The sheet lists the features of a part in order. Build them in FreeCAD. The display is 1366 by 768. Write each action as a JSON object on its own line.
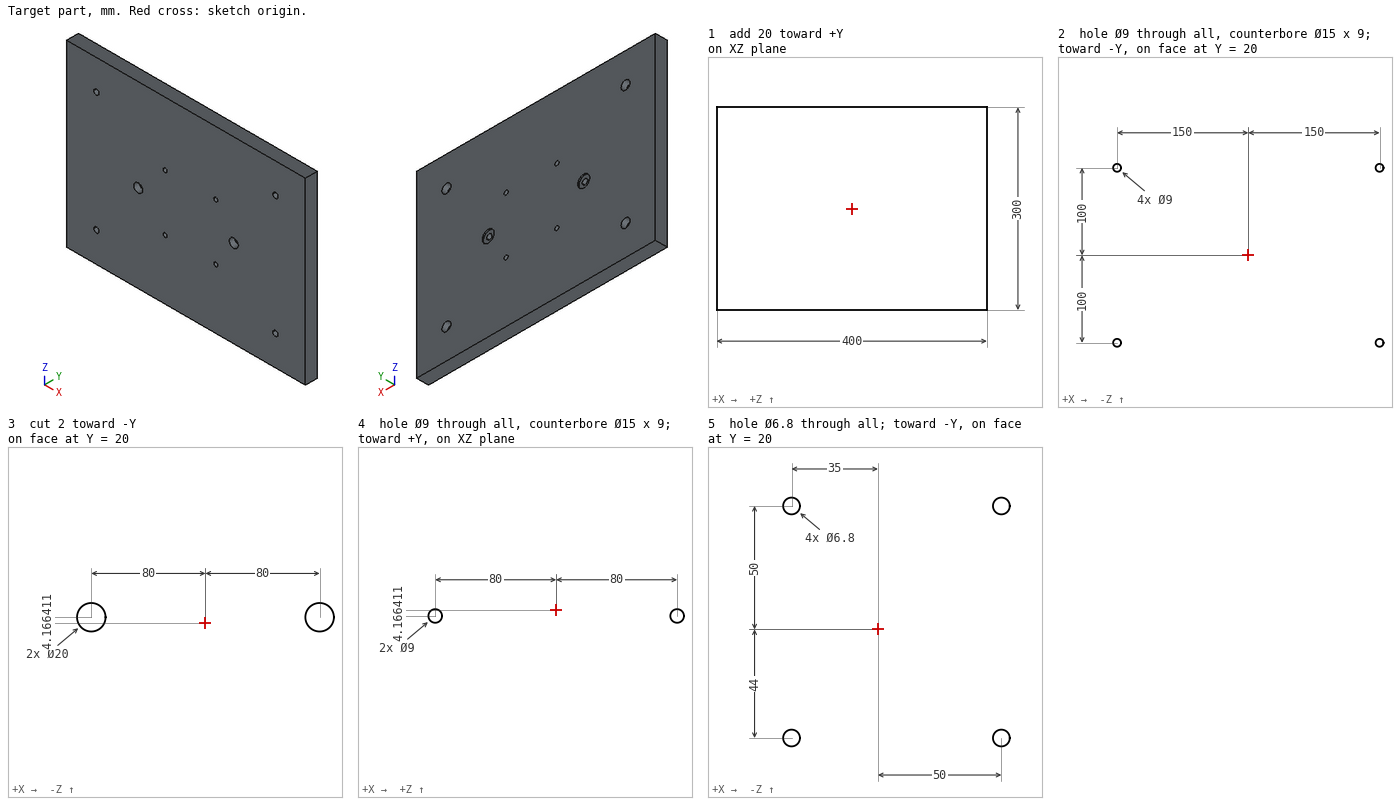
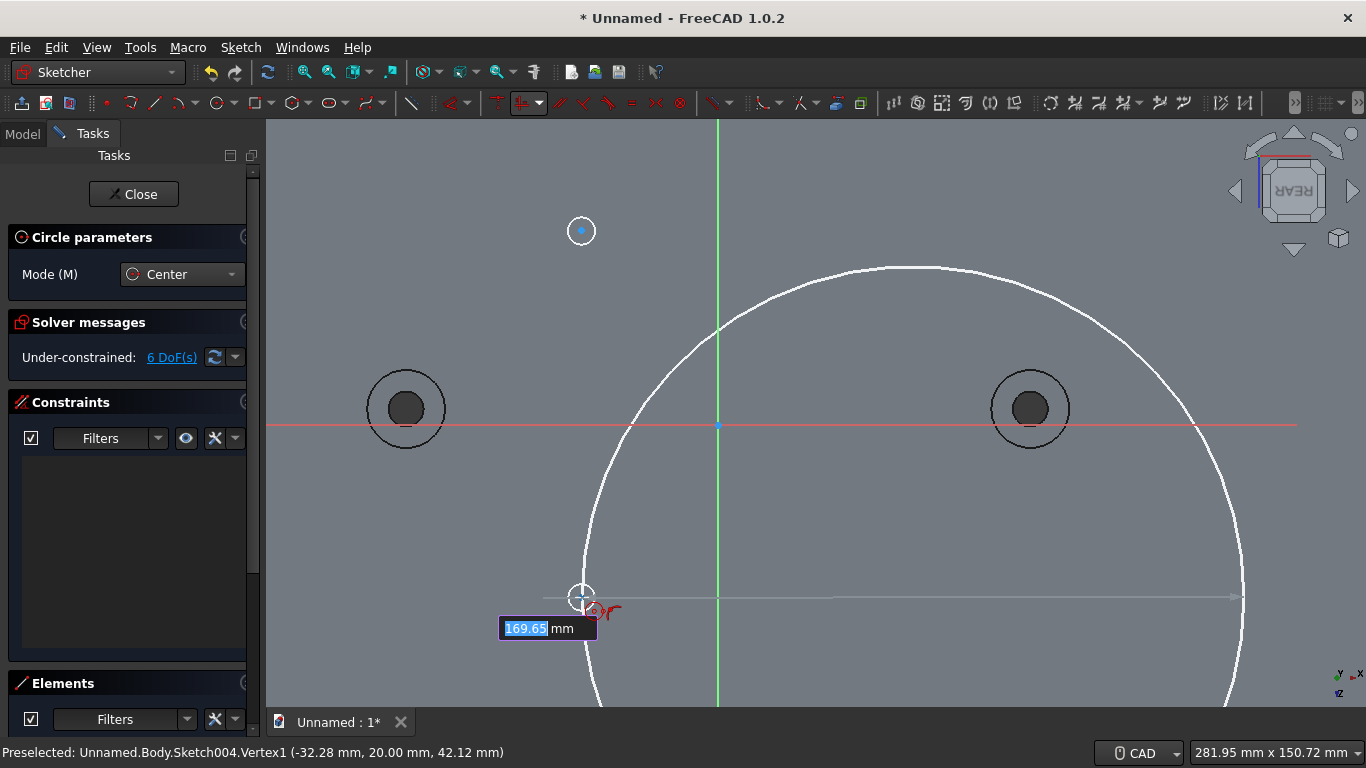
{"action": "left_click", "coordinate": [923, 588]}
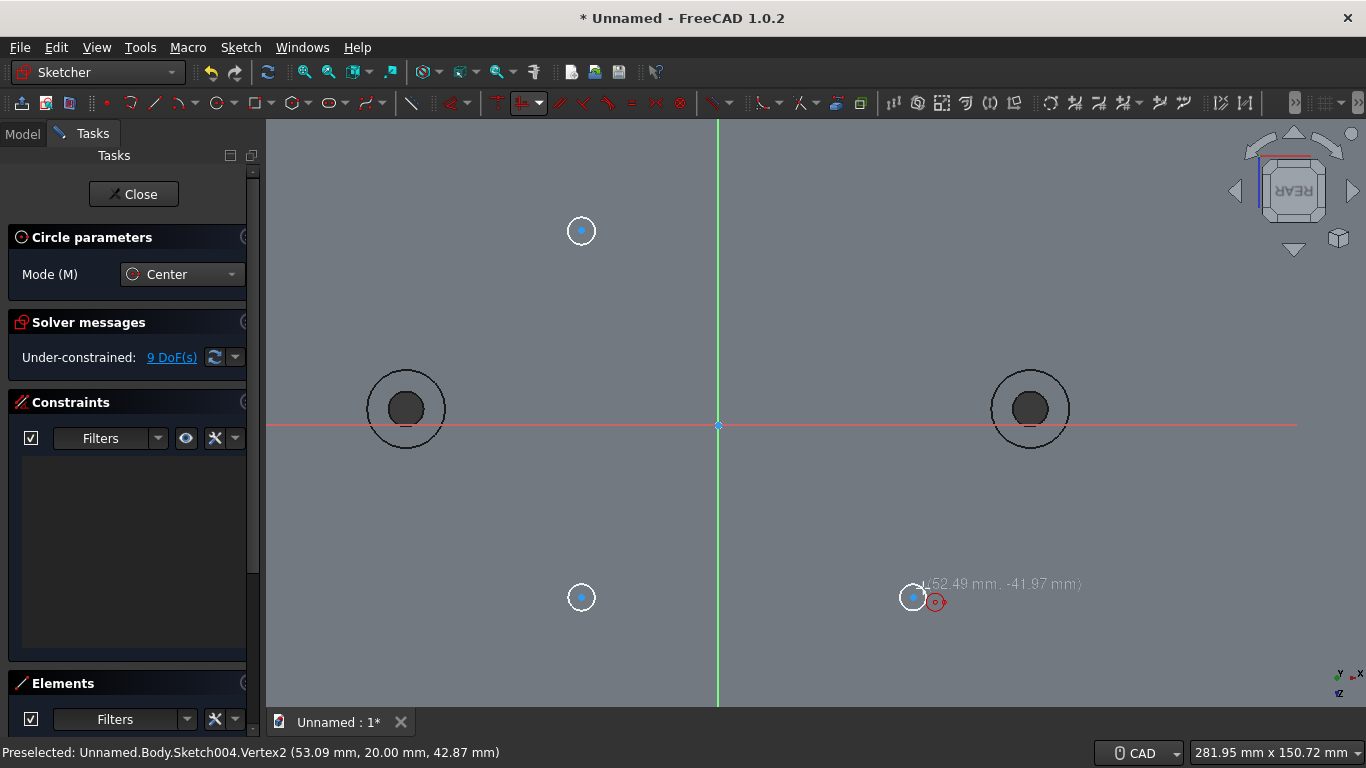
{"action": "scroll", "coordinate": [913, 230], "scroll_direction": "up", "scroll_amount": 3}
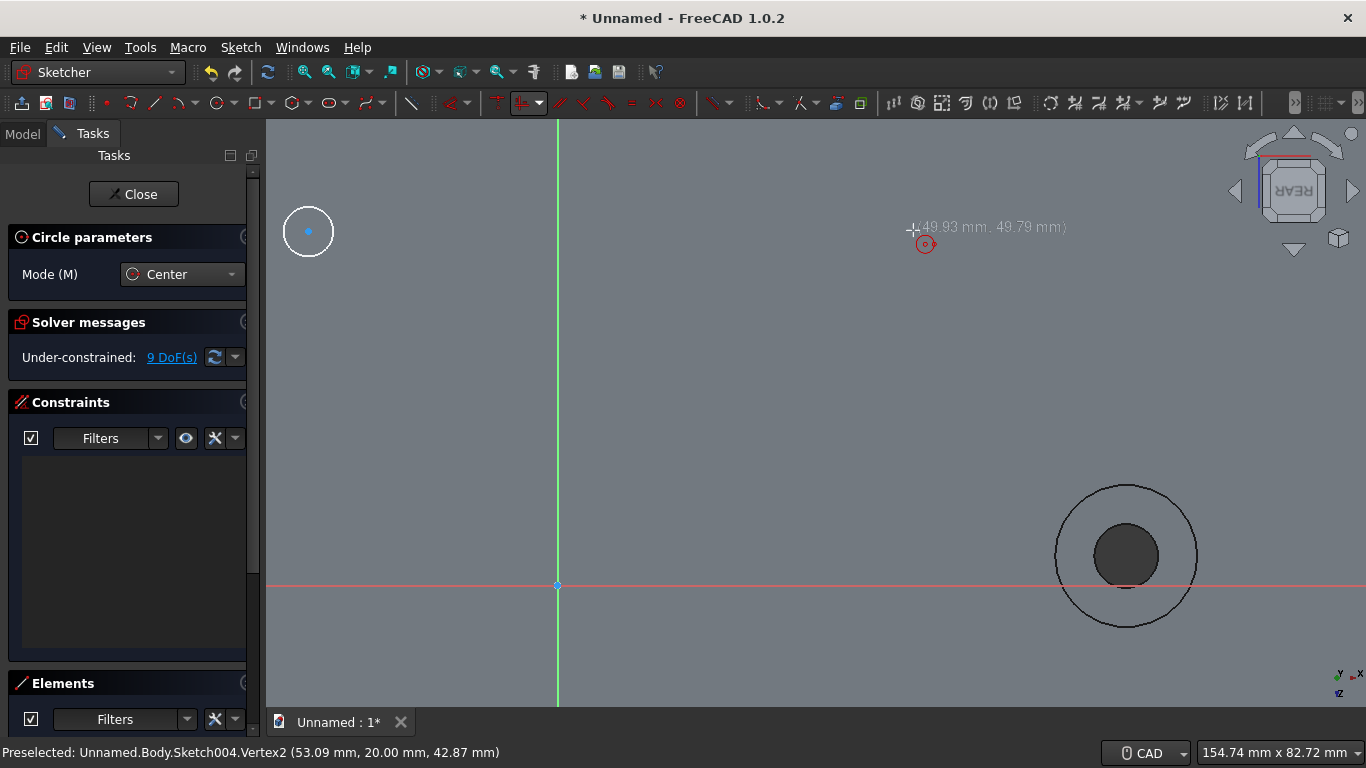
{"action": "left_click", "coordinate": [913, 230]}
{"action": "left_click", "coordinate": [930, 213]}
{"action": "key", "text": "Escape"}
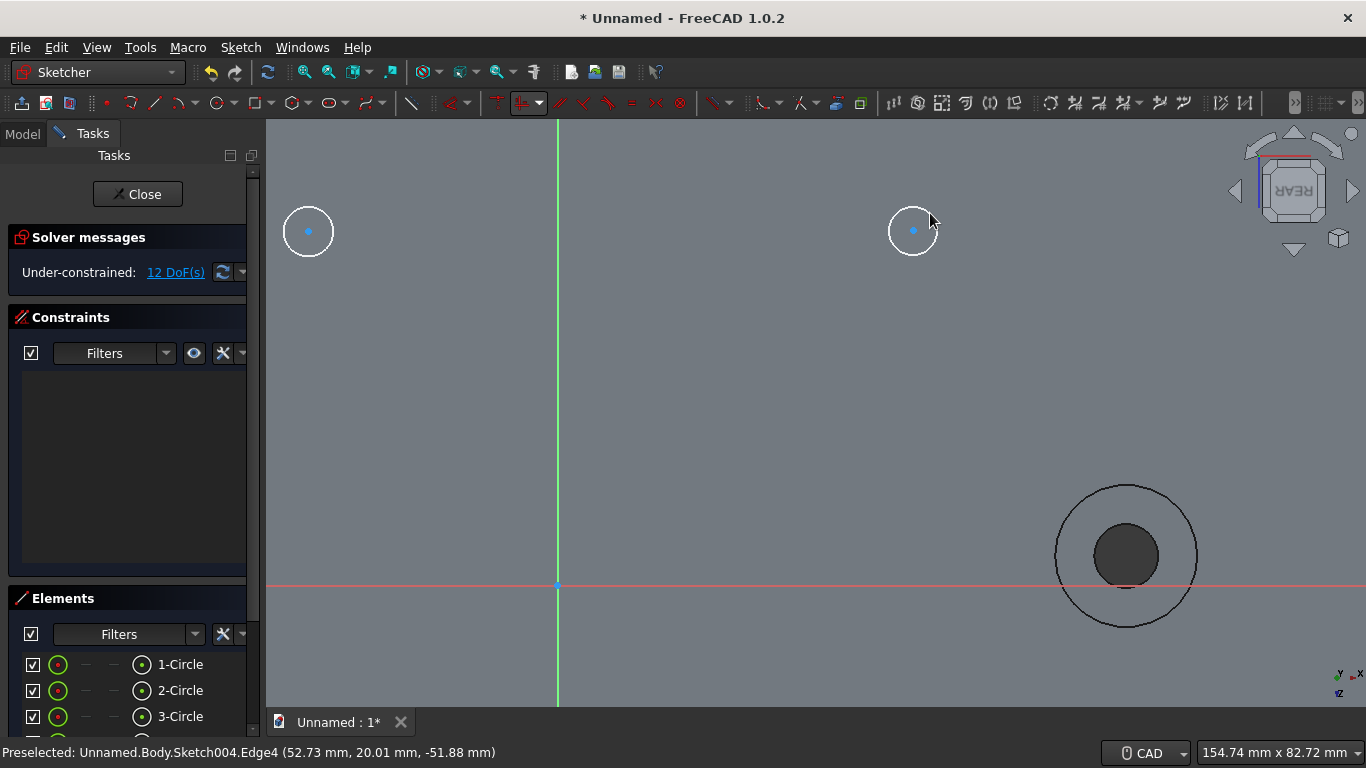
{"action": "left_click", "coordinate": [326, 214]}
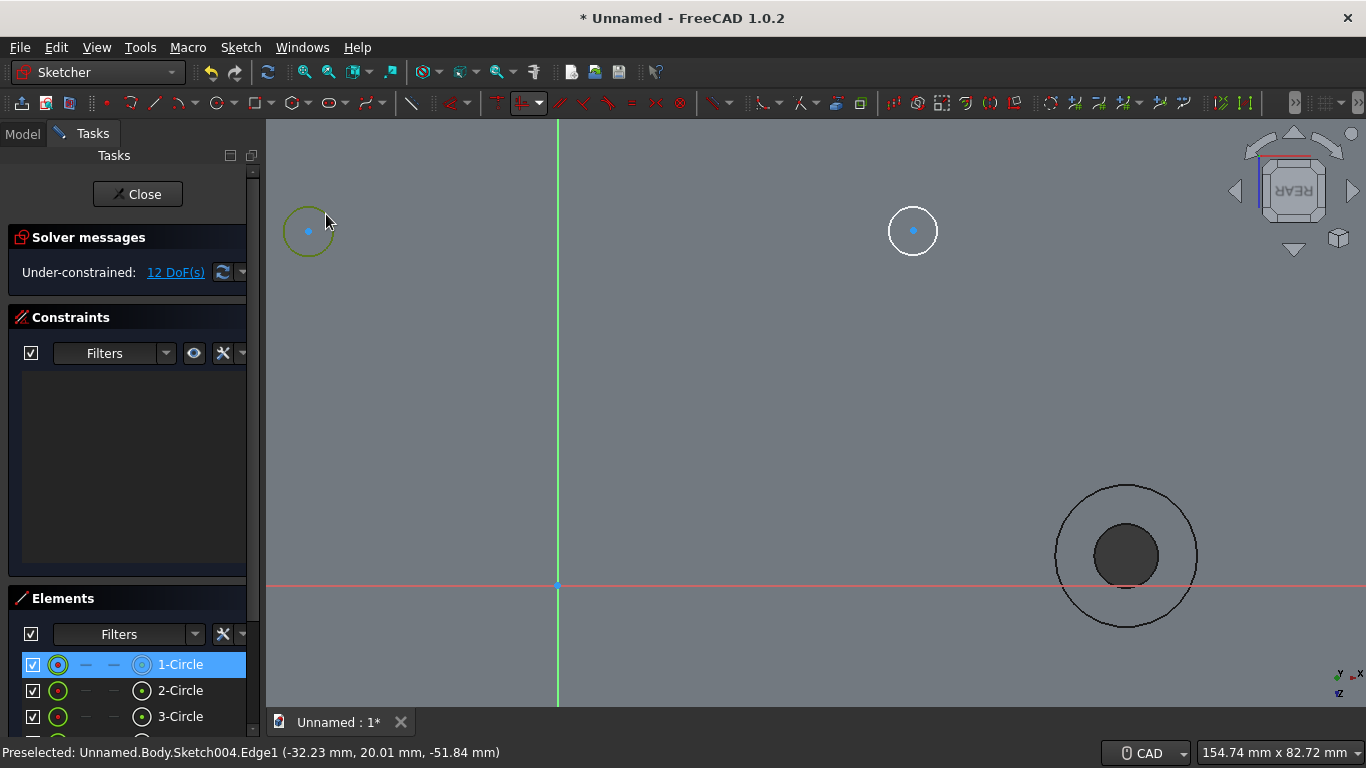
{"action": "scroll", "coordinate": [914, 229], "scroll_direction": "down", "scroll_amount": 3}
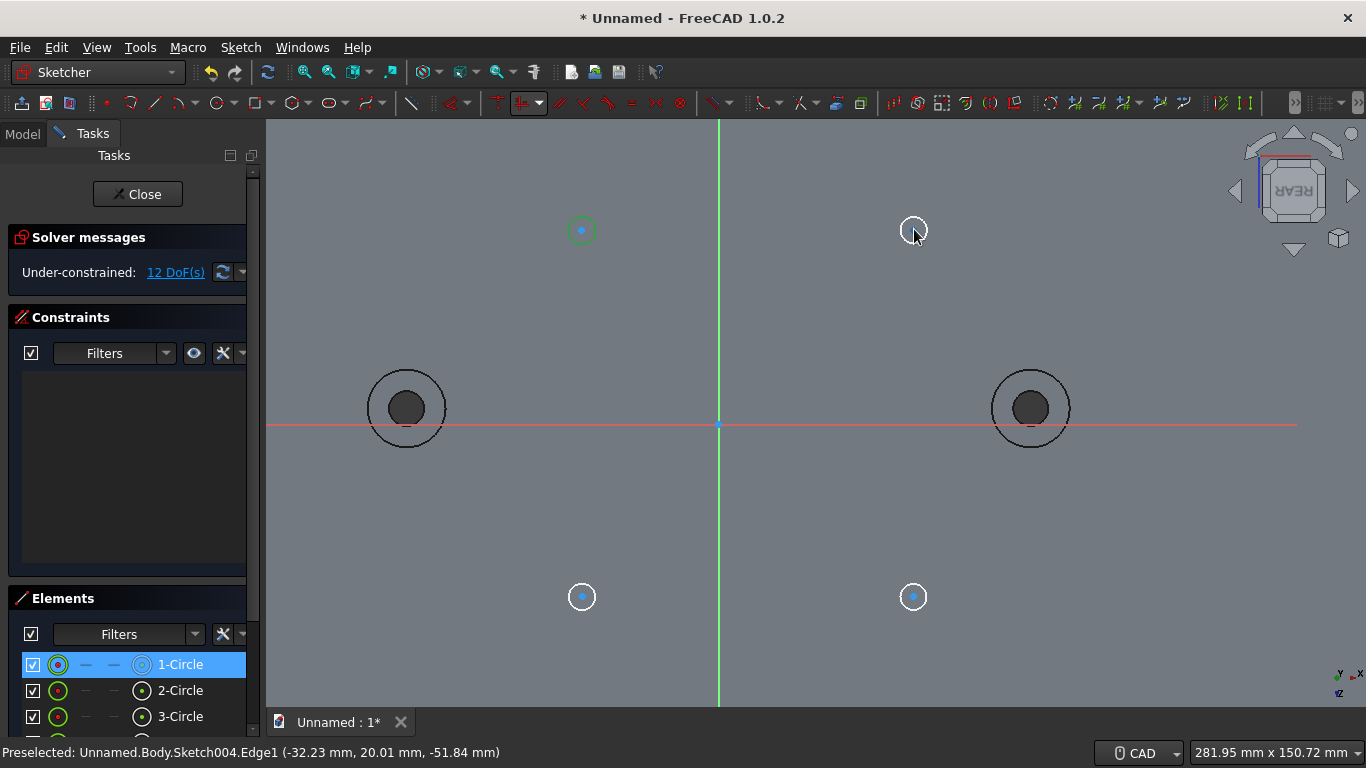
{"action": "left_click", "coordinate": [591, 588]}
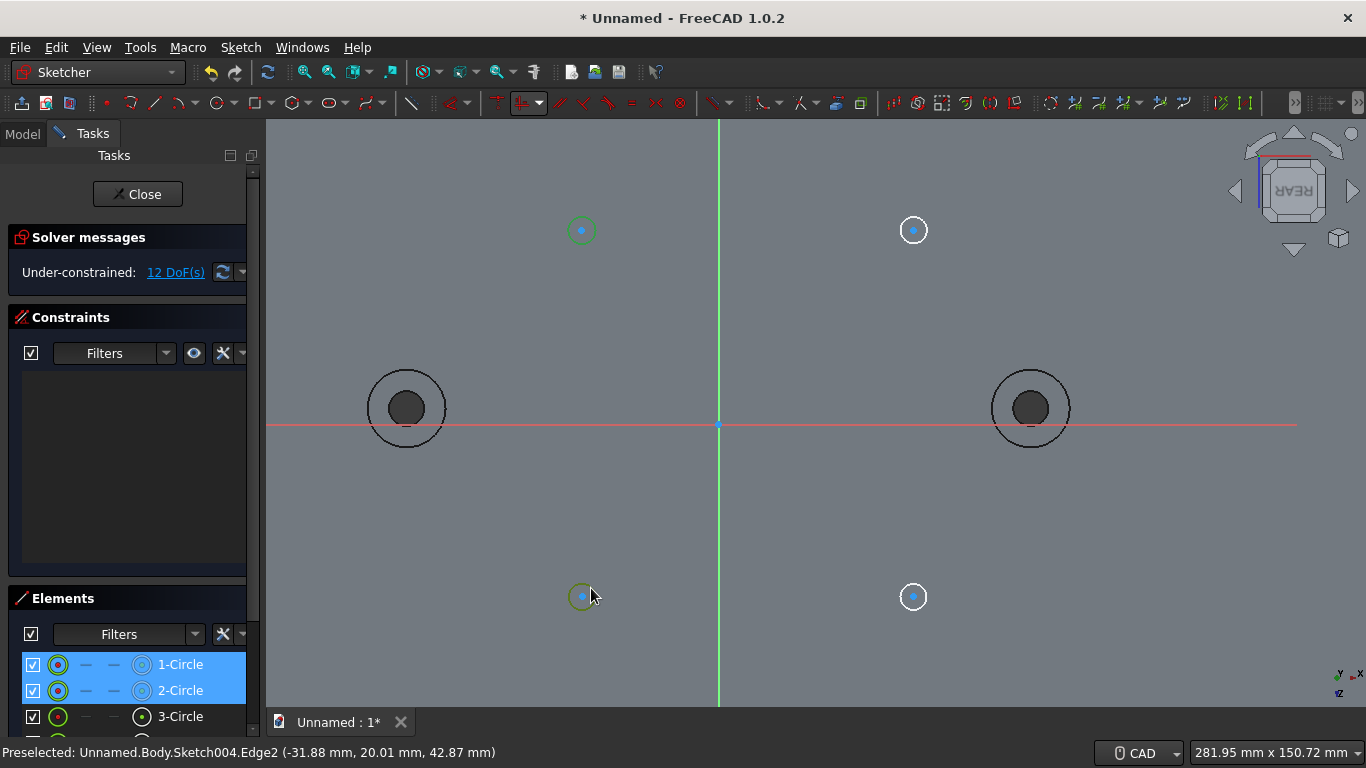
{"action": "left_click", "coordinate": [923, 588]}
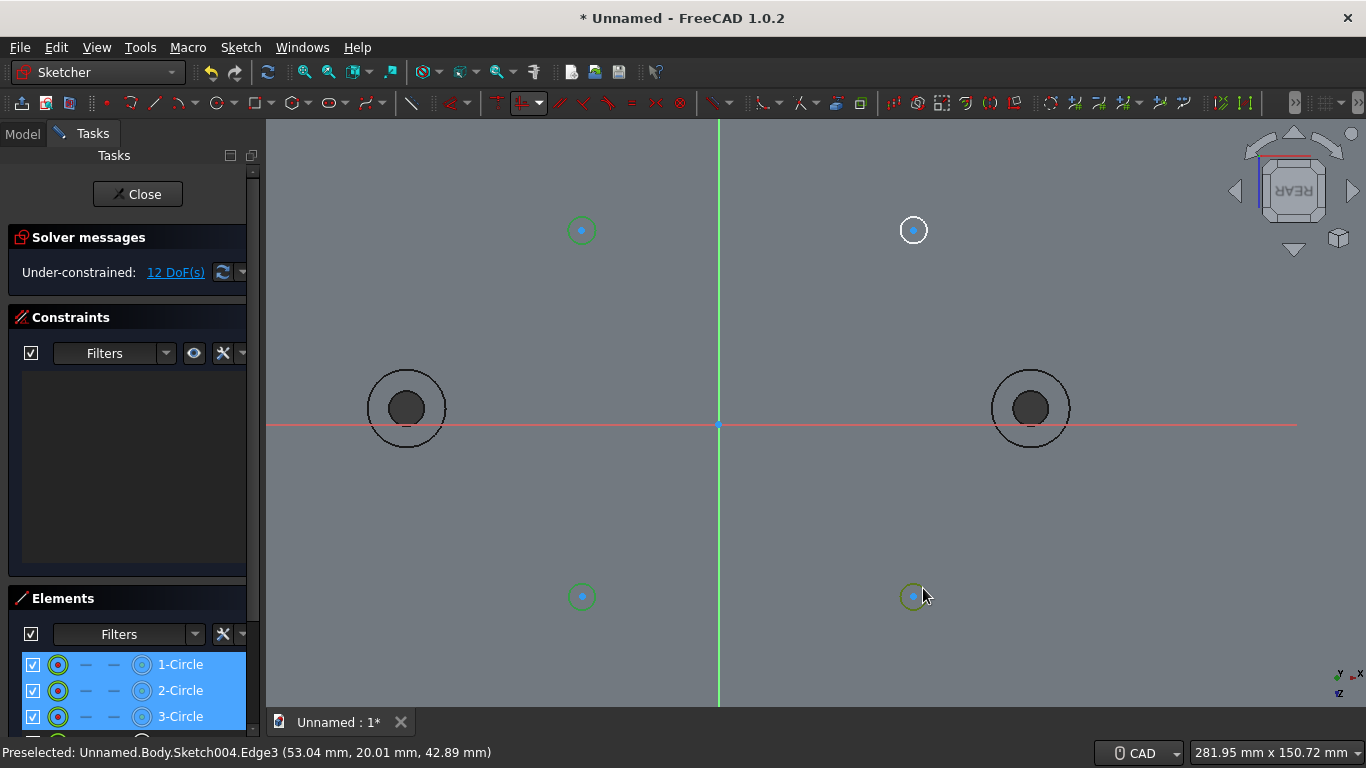
{"action": "left_click", "coordinate": [923, 221]}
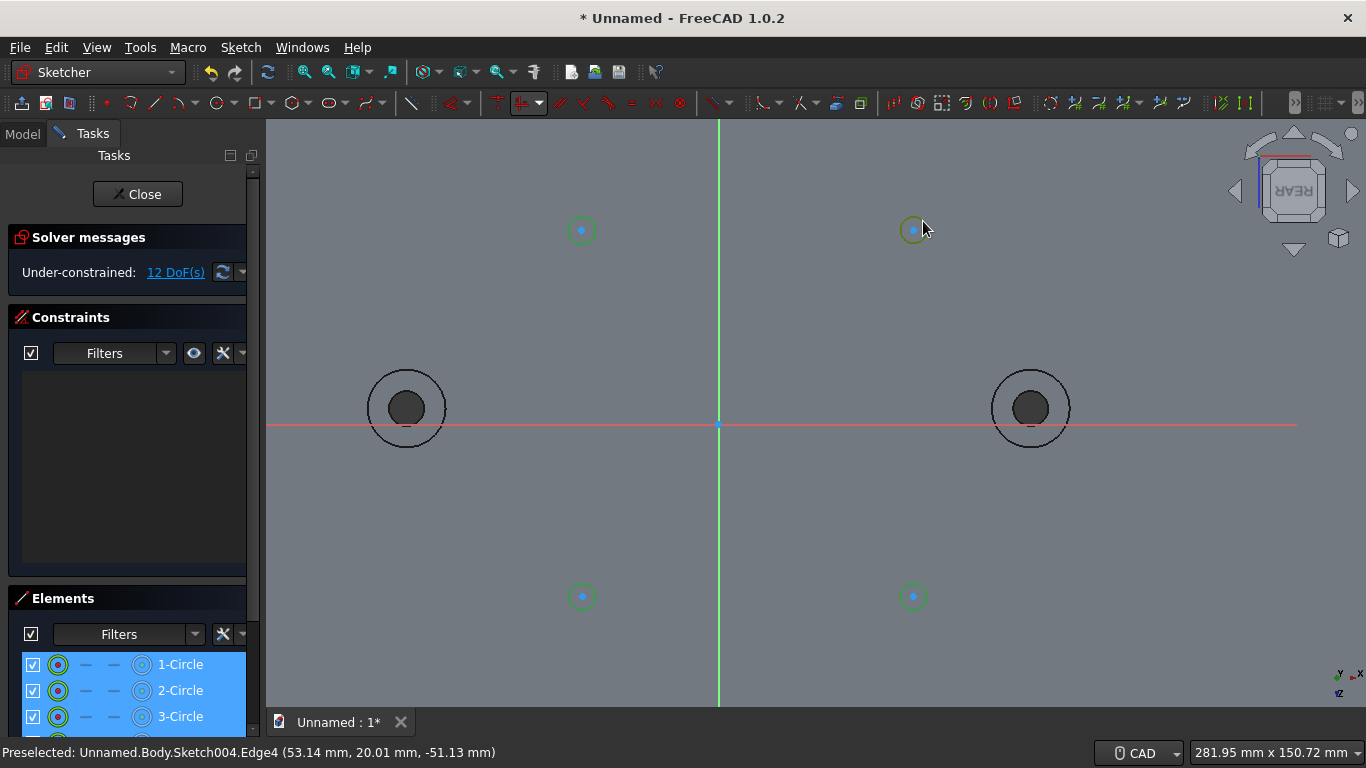
{"action": "key", "text": "e"}